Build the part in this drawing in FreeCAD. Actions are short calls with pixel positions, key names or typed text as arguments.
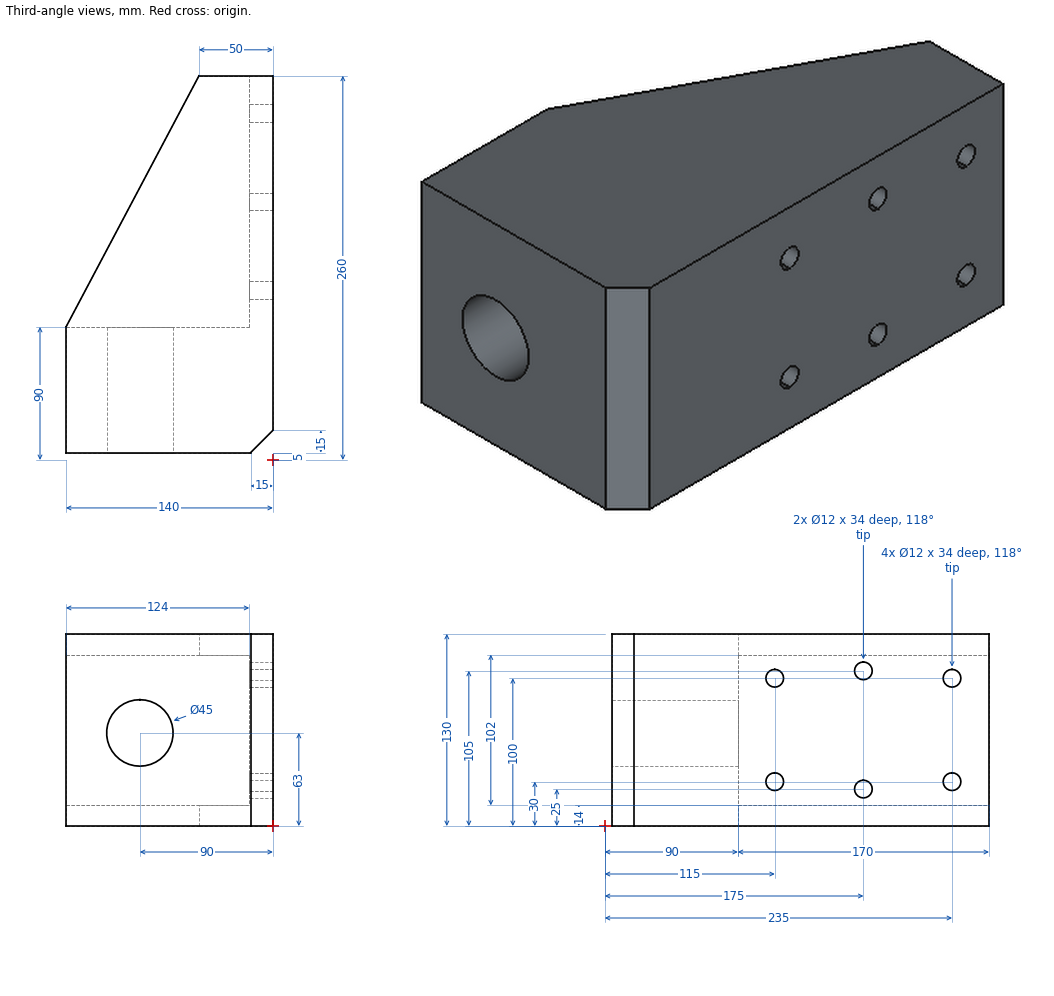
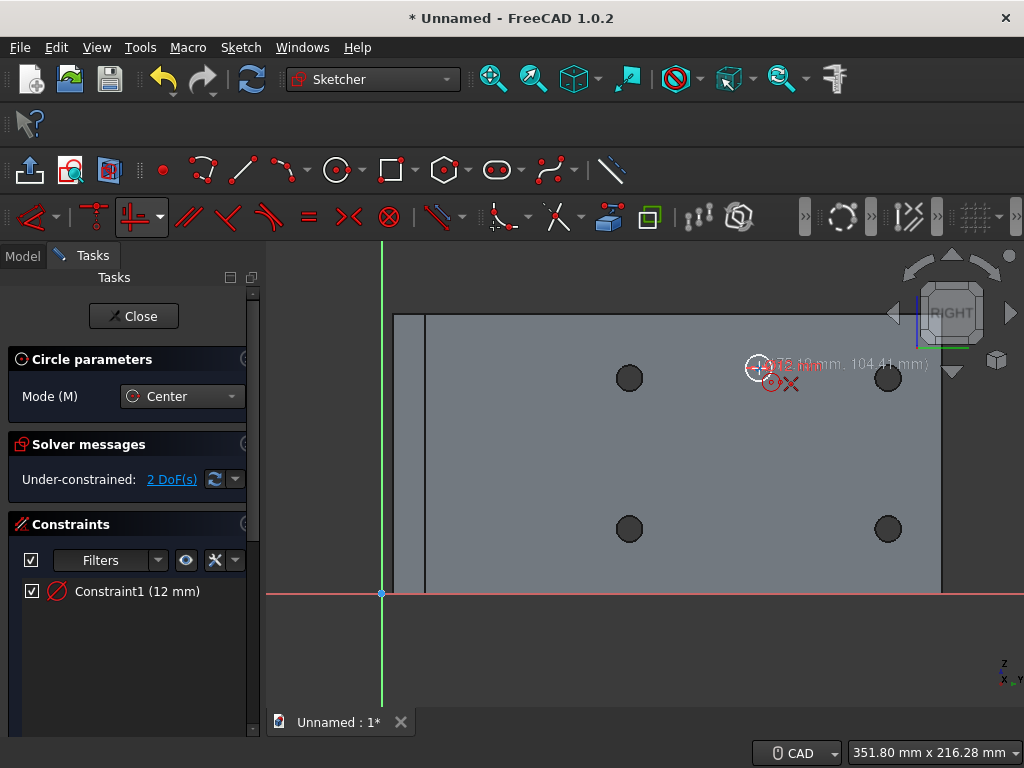
scroll(759, 540, up, 3)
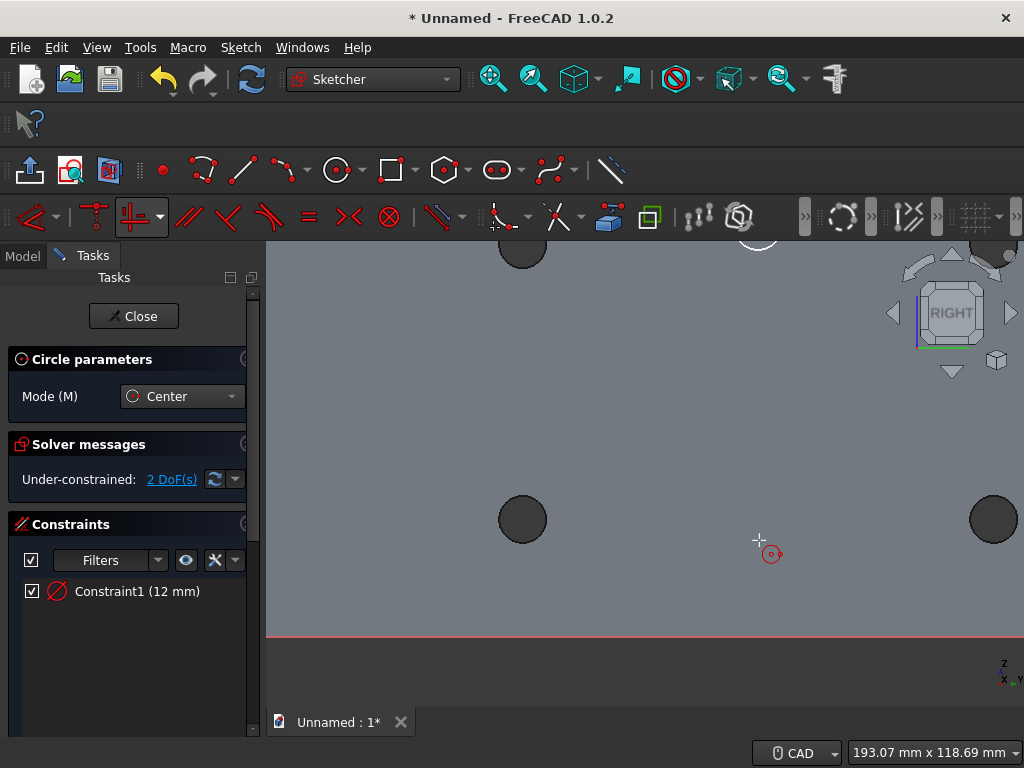
click(758, 539)
move(775, 522)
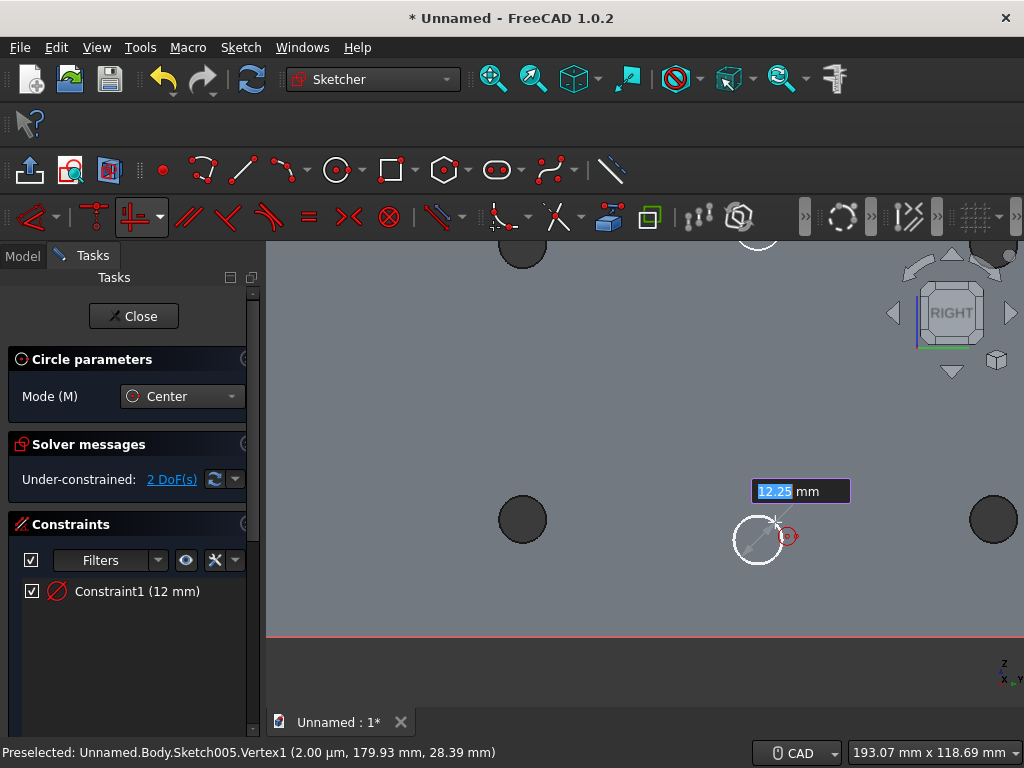
text(12)
key(Return)
key(Escape)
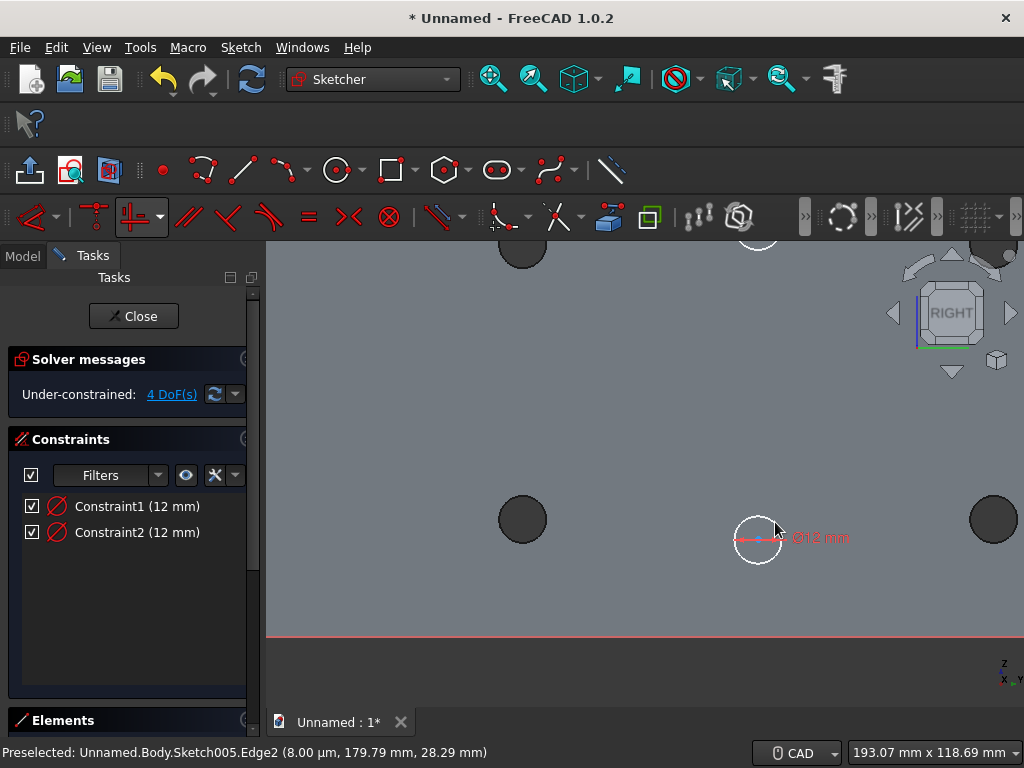
scroll(759, 541, down, 3)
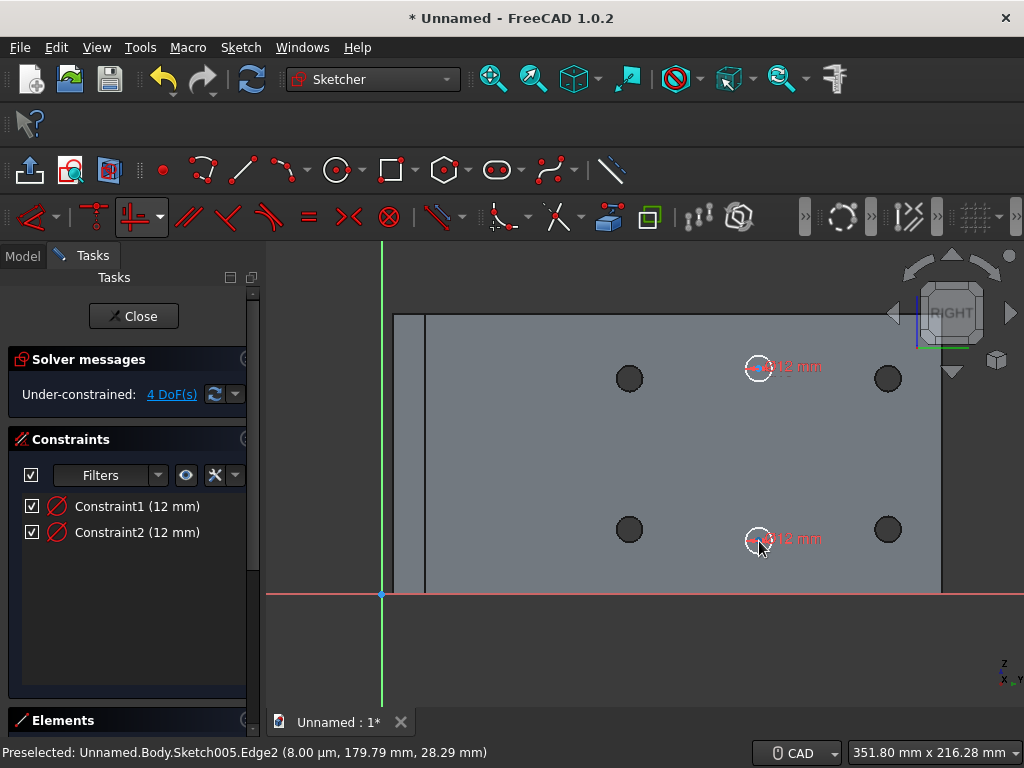
click(759, 369)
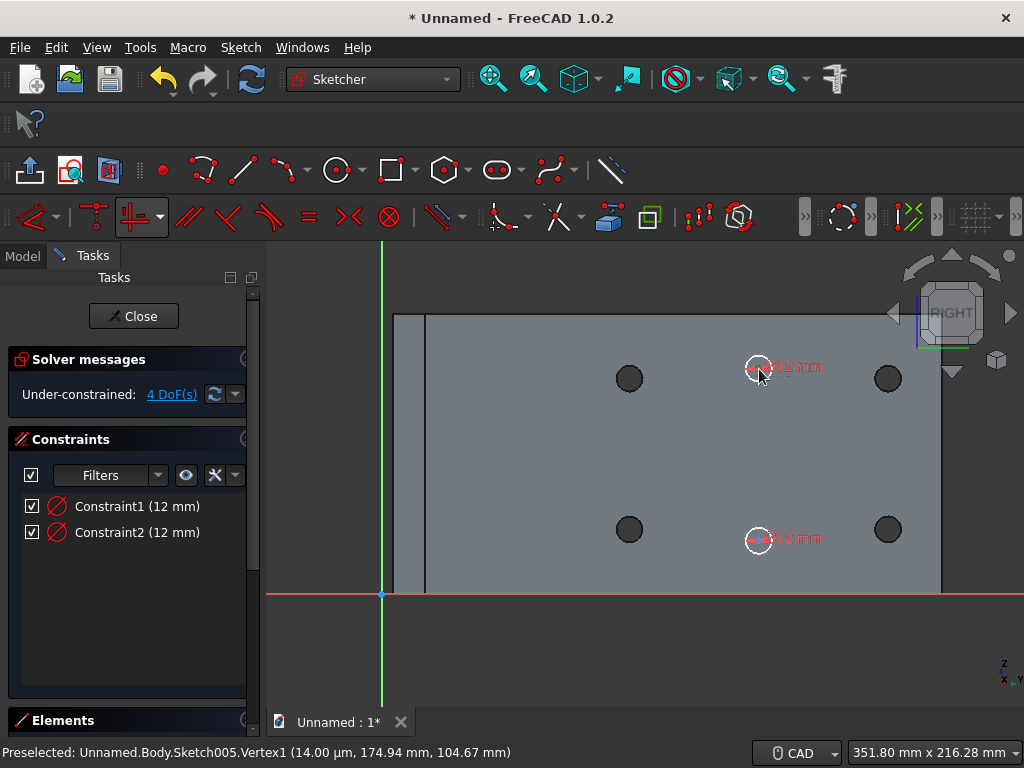
click(759, 541)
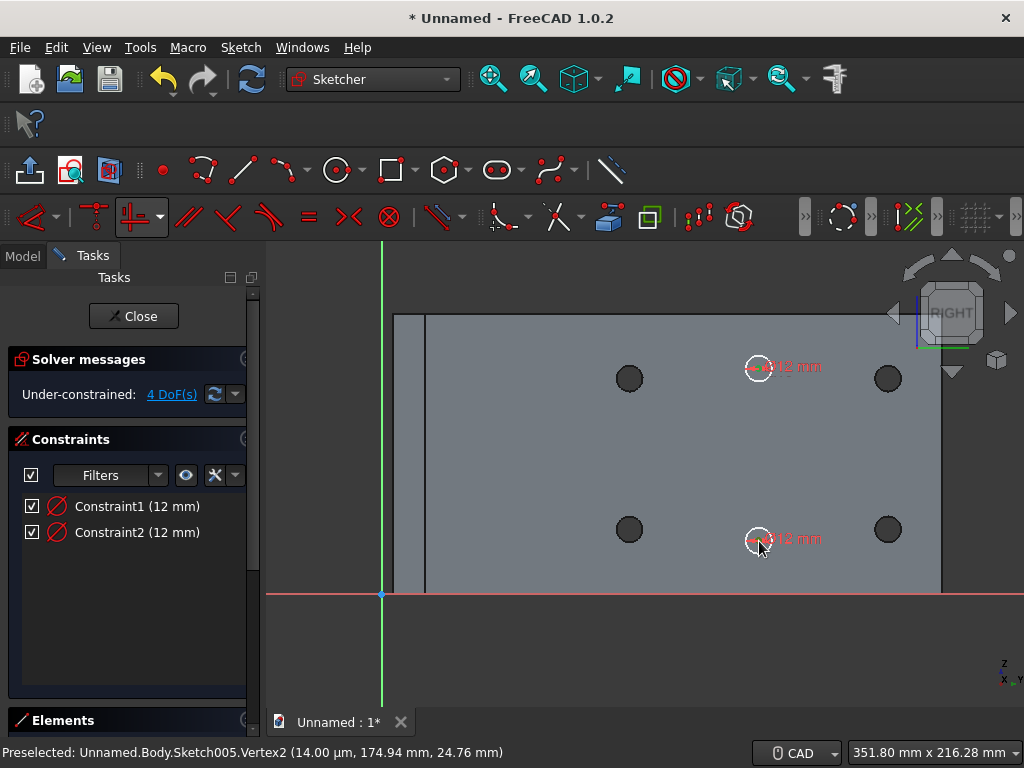
click(162, 218)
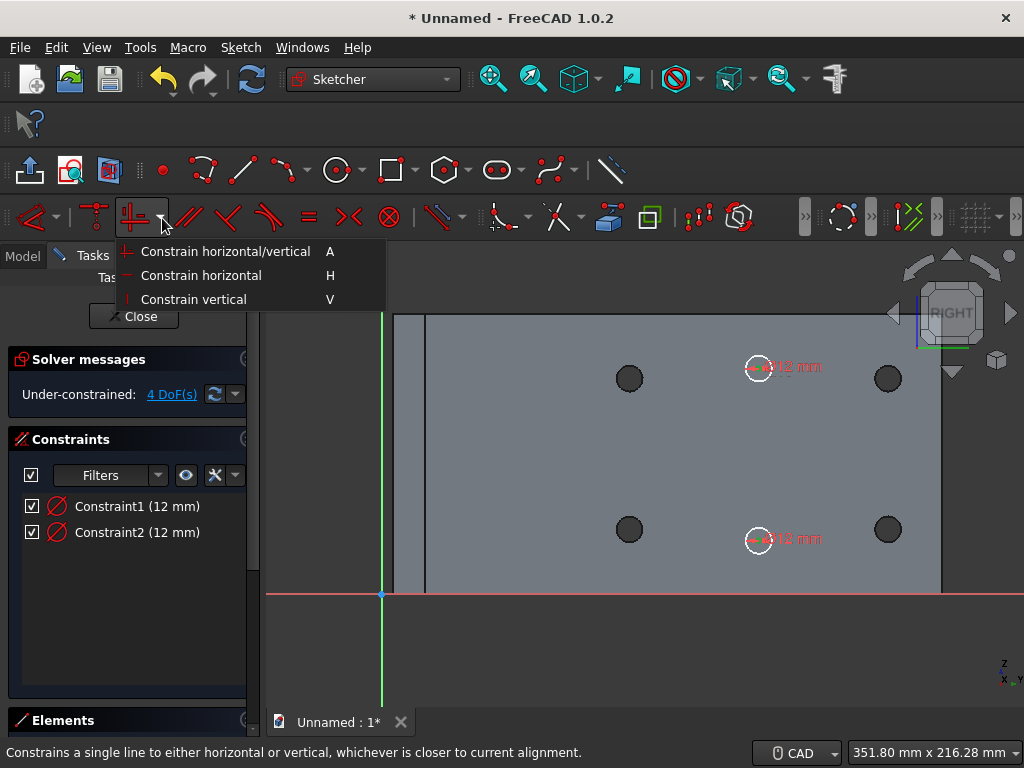
click(251, 299)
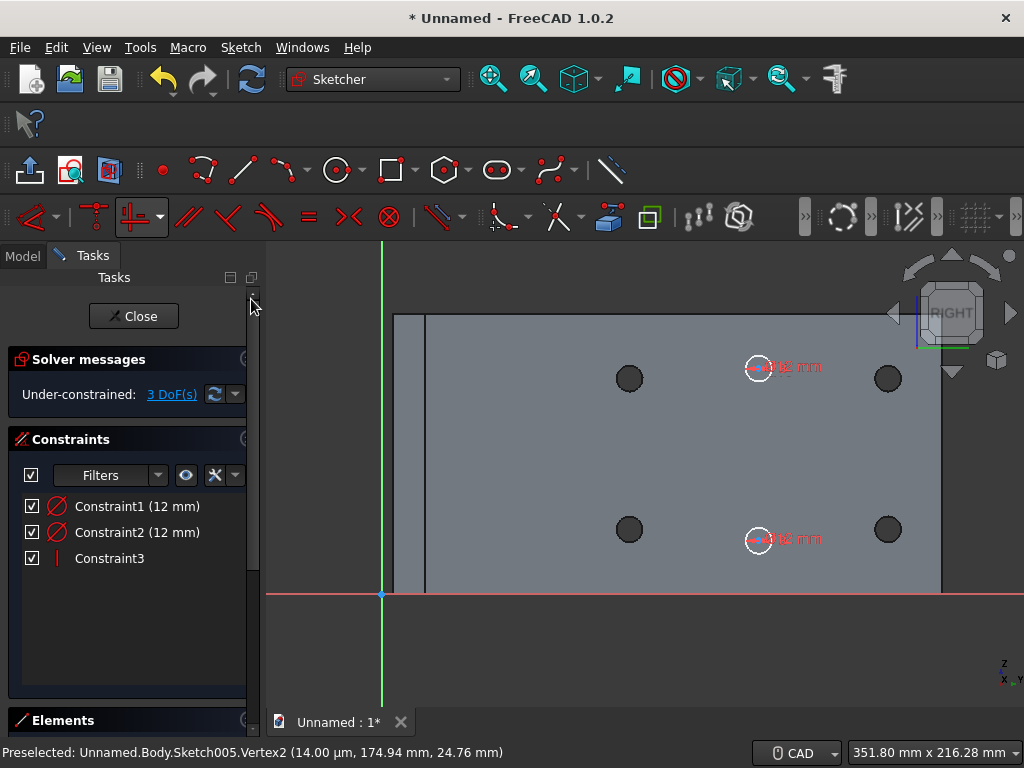
click(32, 218)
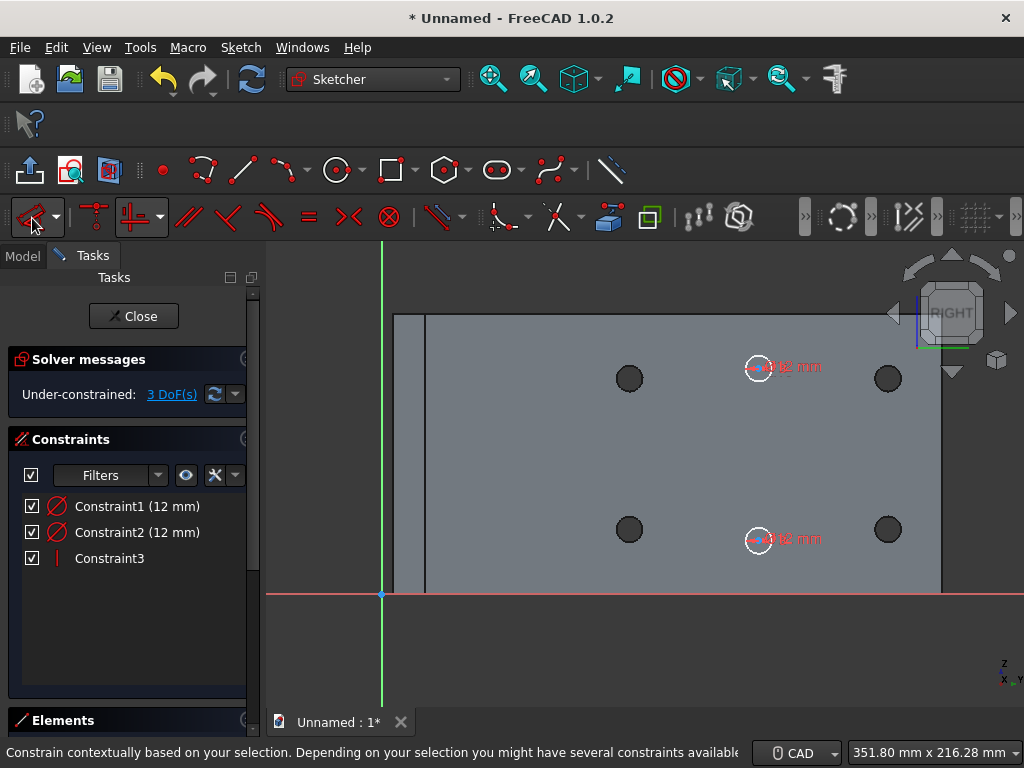
click(759, 541)
click(348, 567)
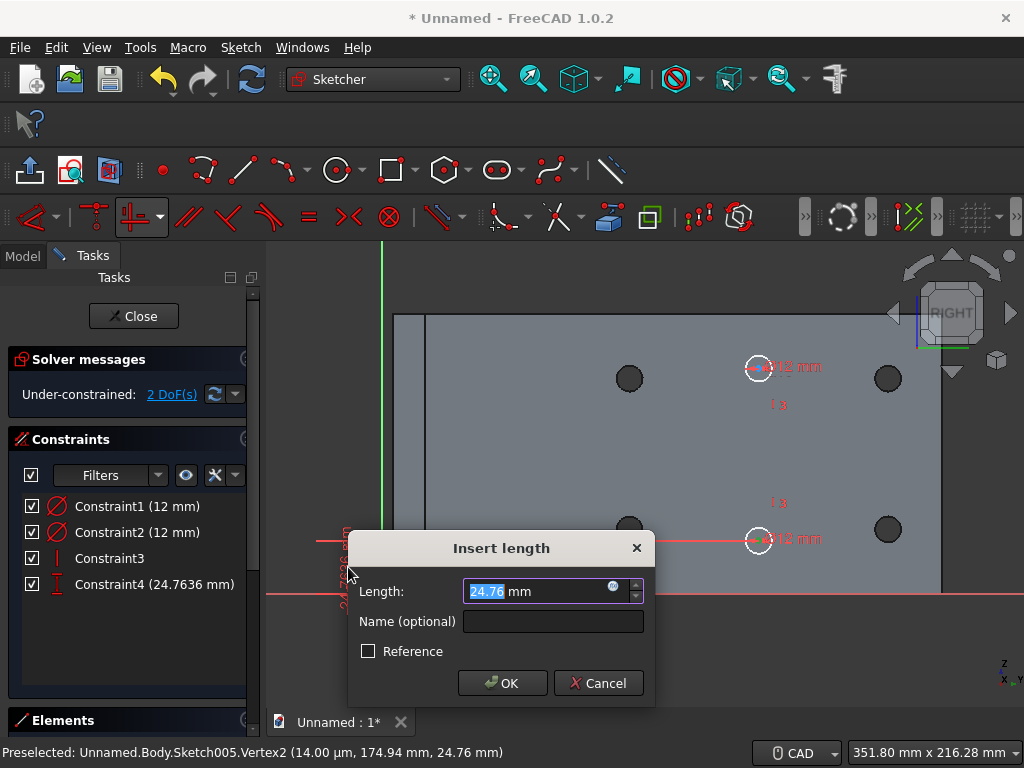
text(25)
key(Return)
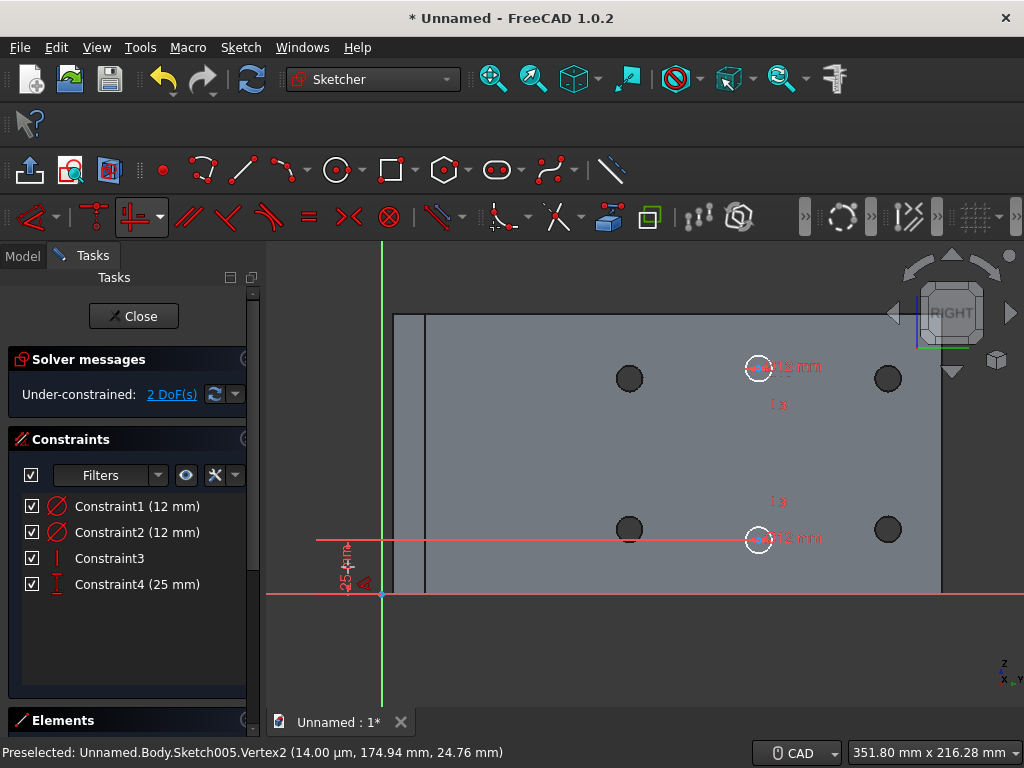
click(759, 369)
click(570, 628)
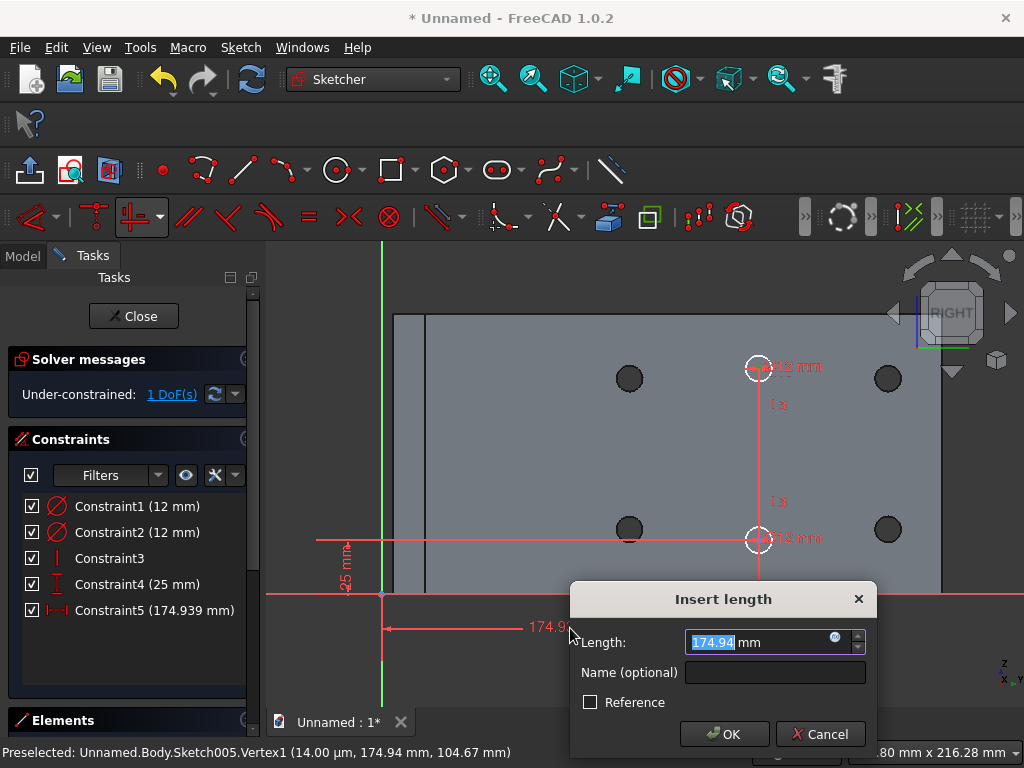
text(175)
key(Return)